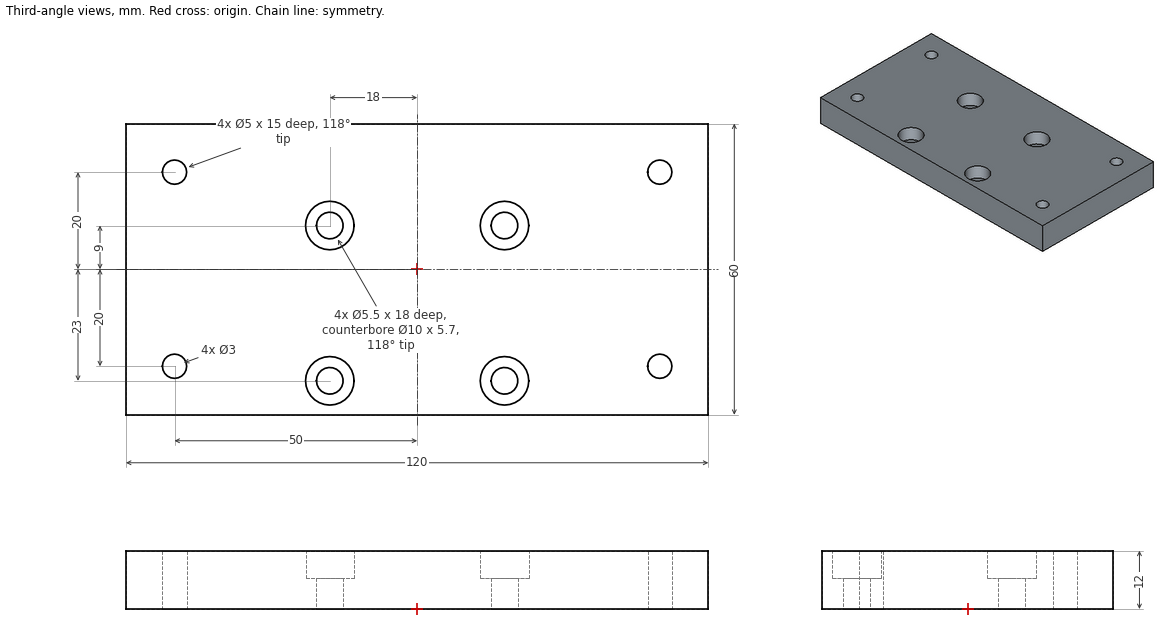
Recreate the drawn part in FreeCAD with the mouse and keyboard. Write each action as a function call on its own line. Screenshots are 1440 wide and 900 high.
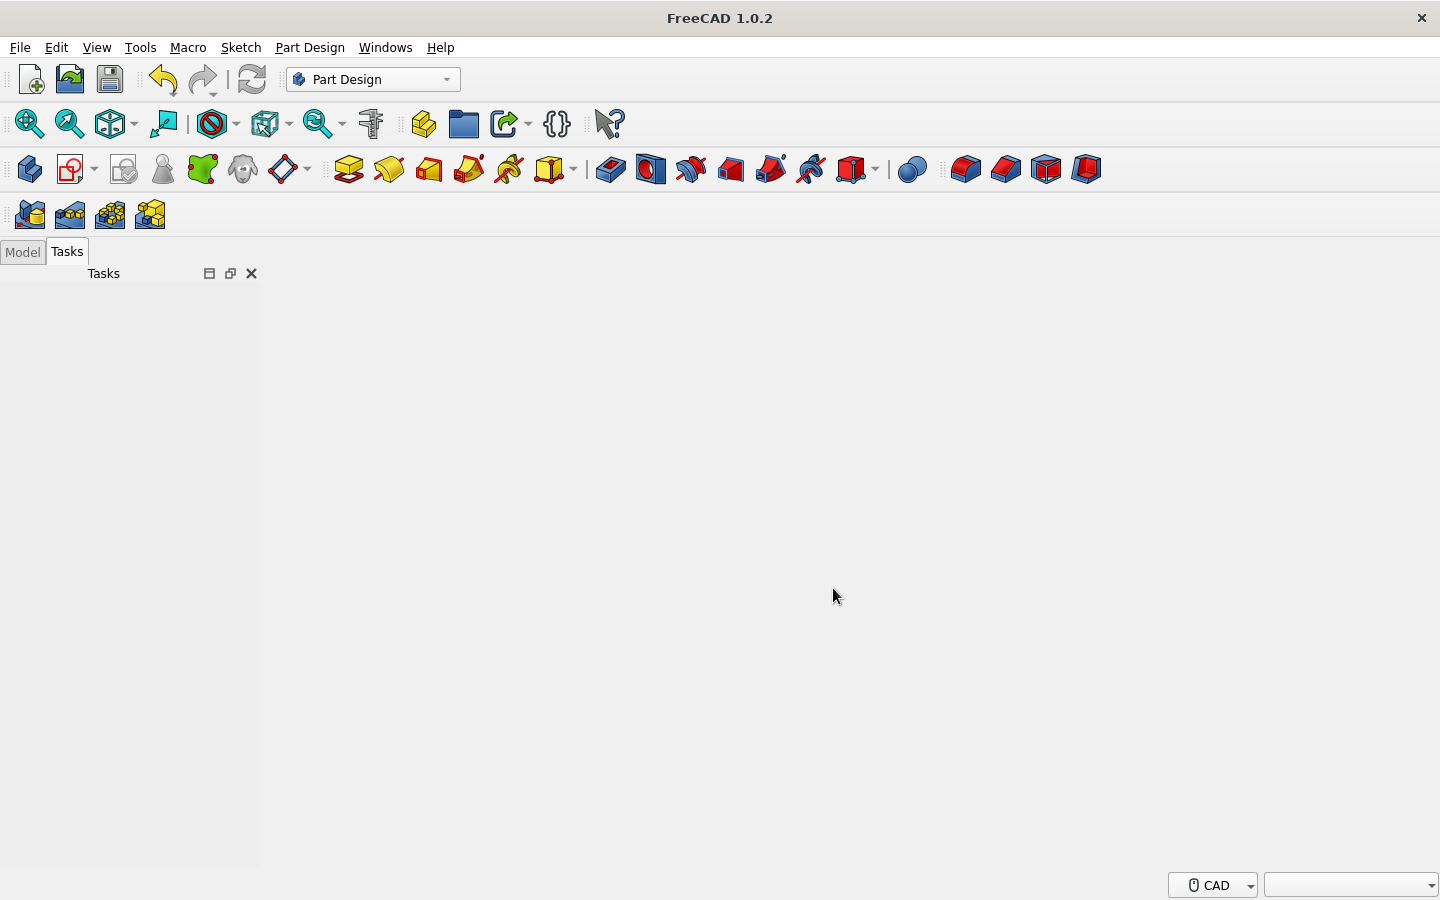
click(30, 80)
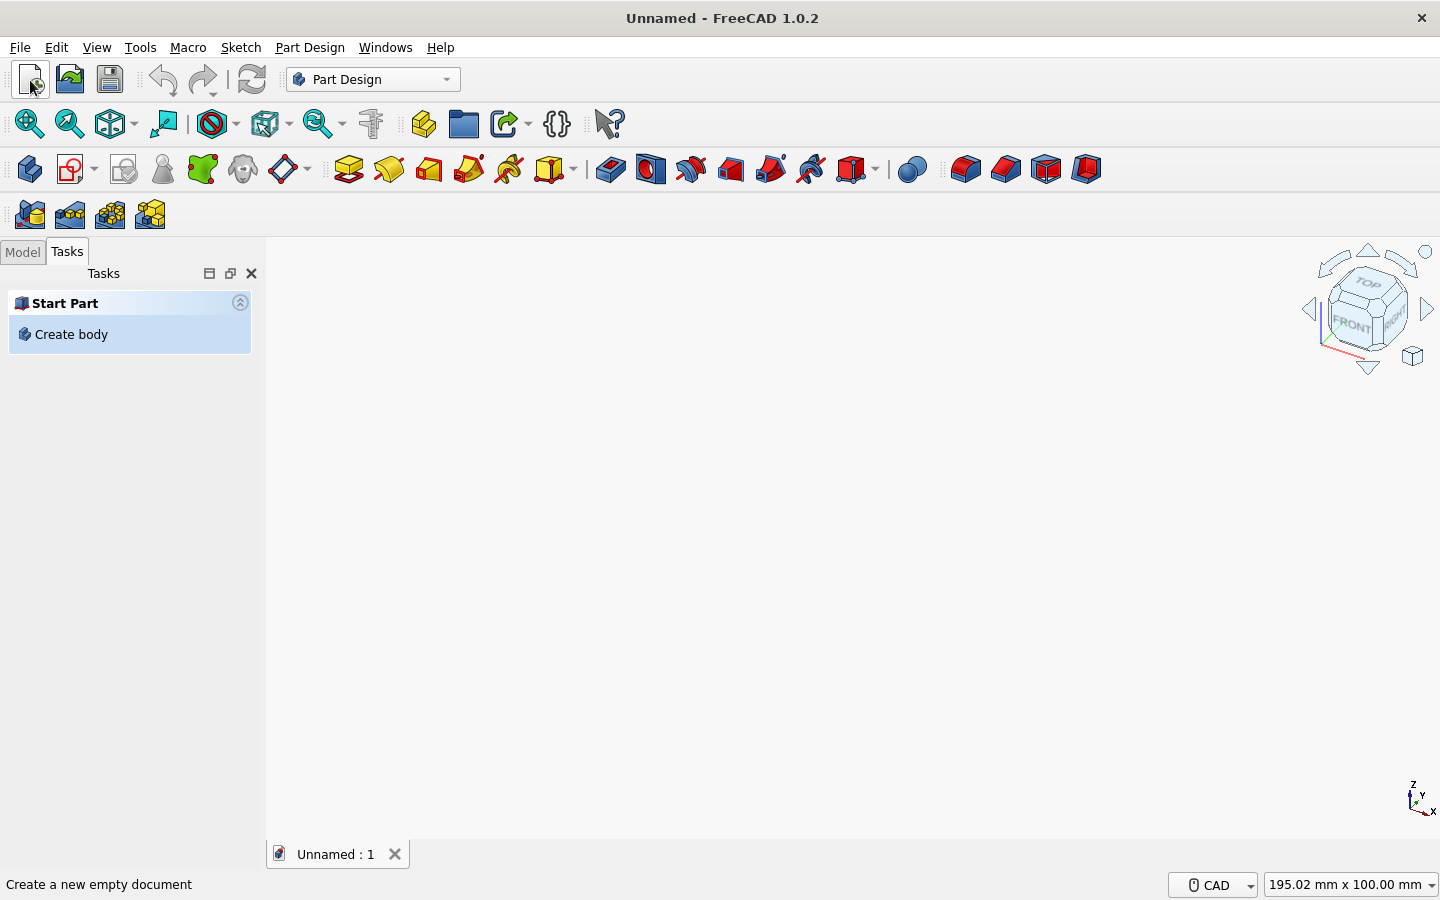
click(70, 170)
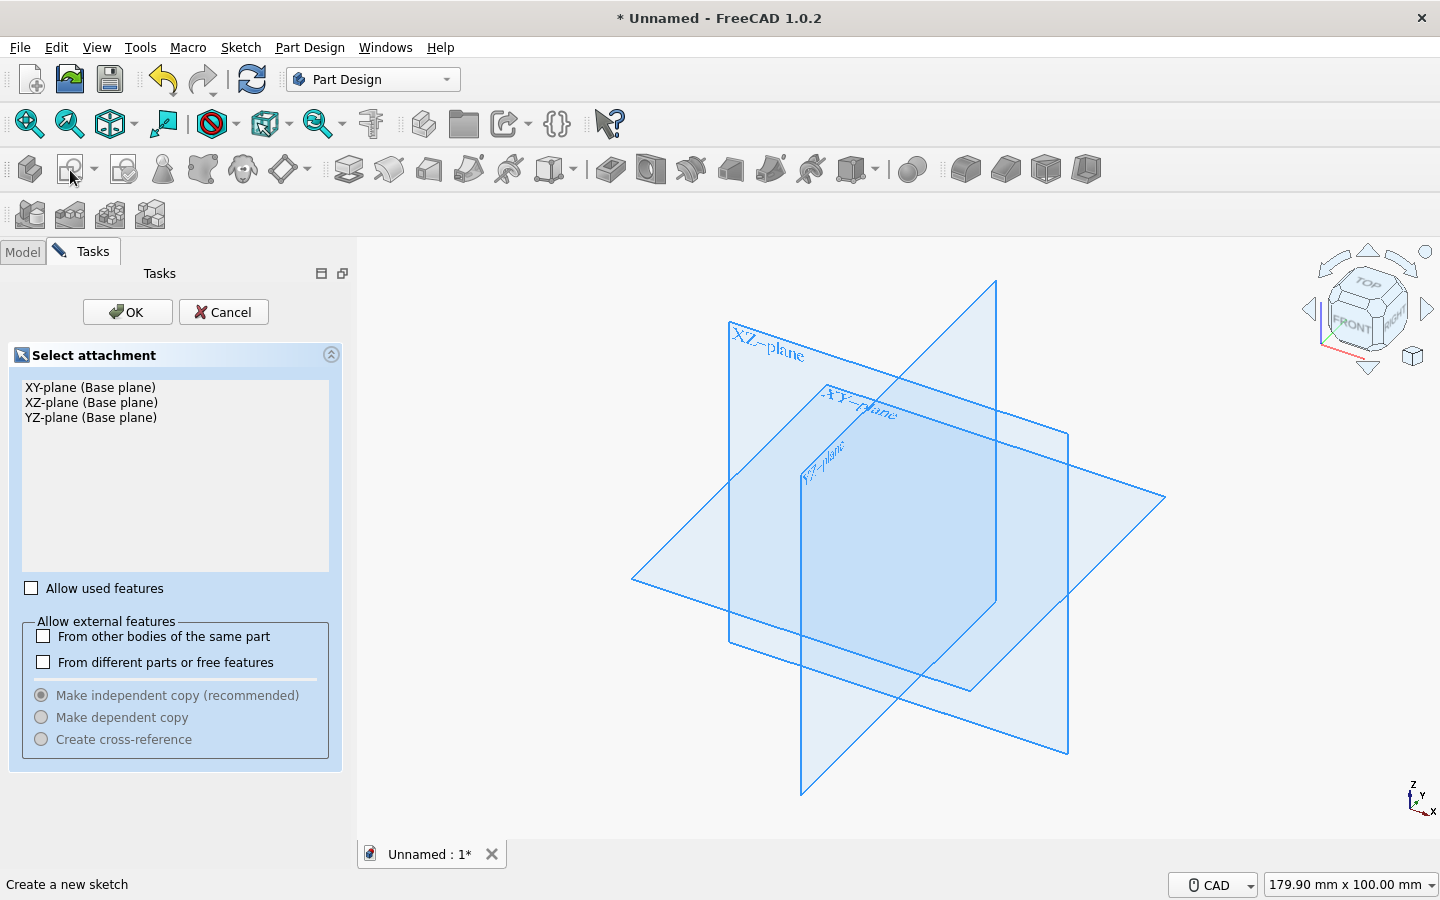
click(82, 388)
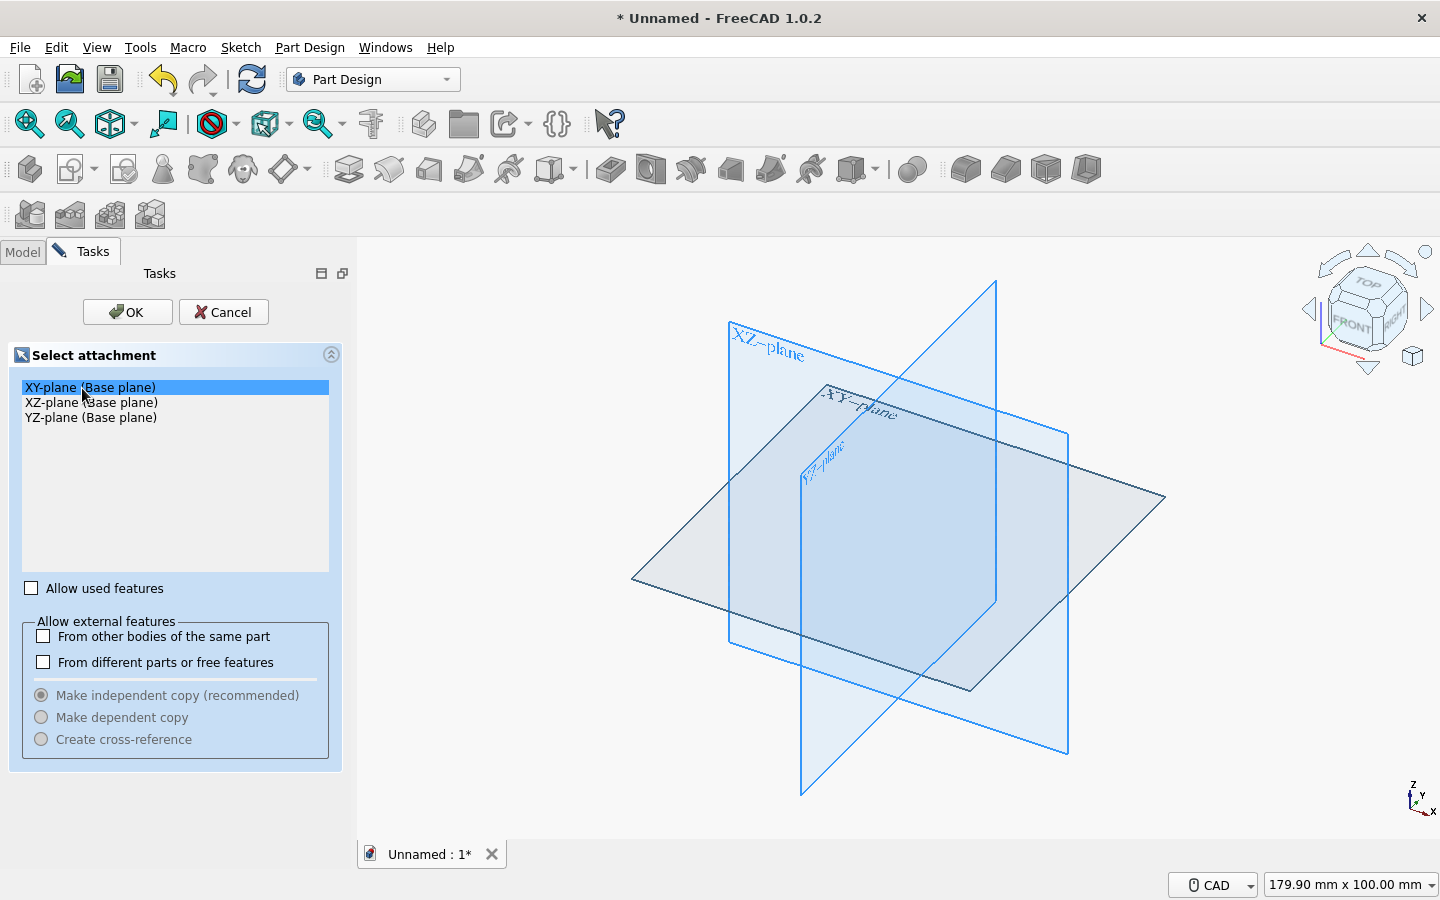
click(128, 312)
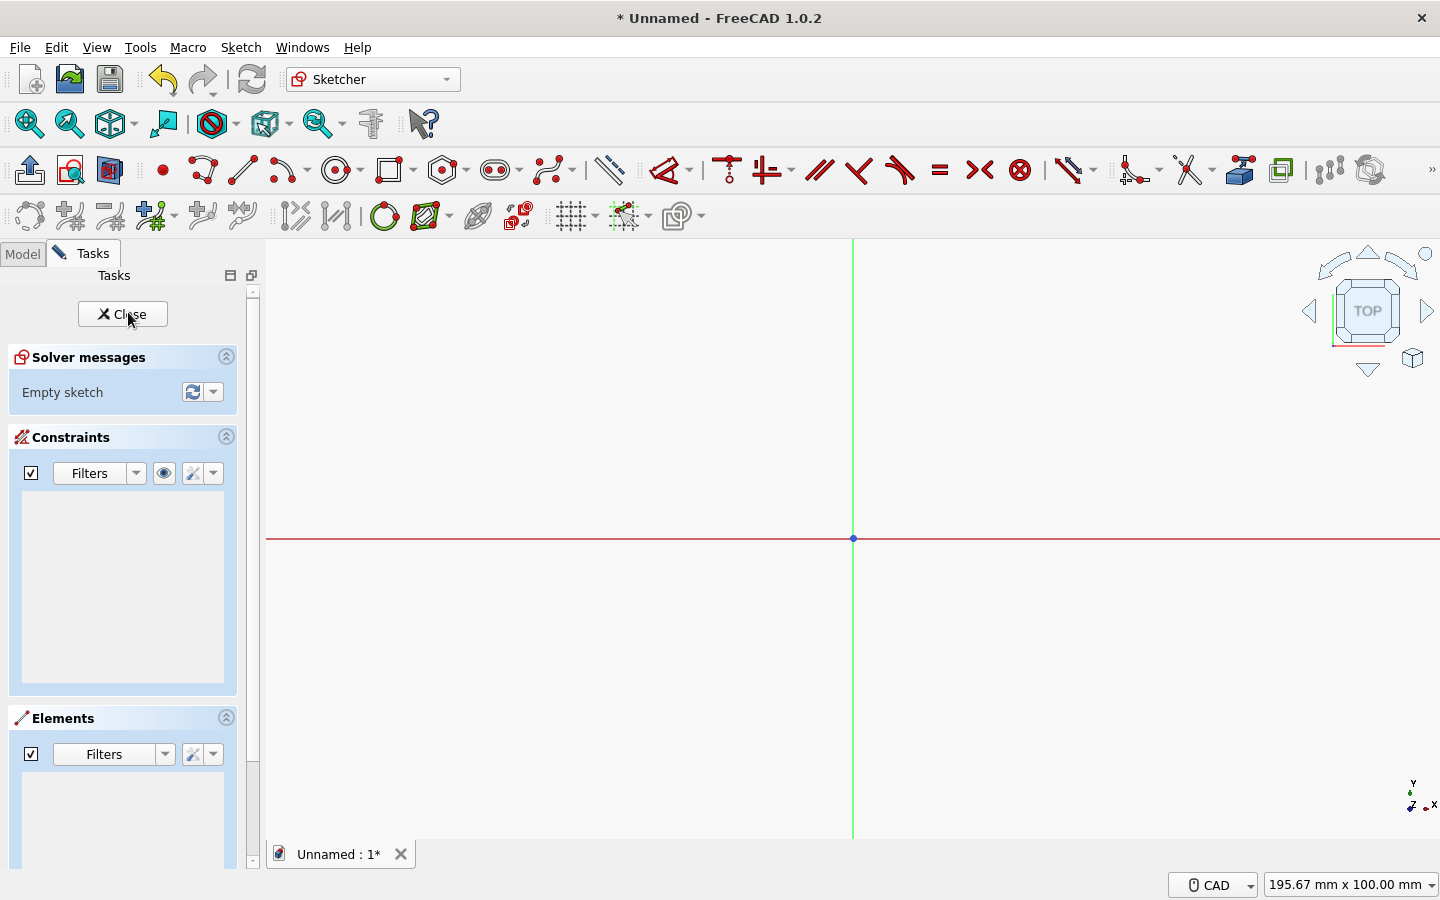
click(416, 170)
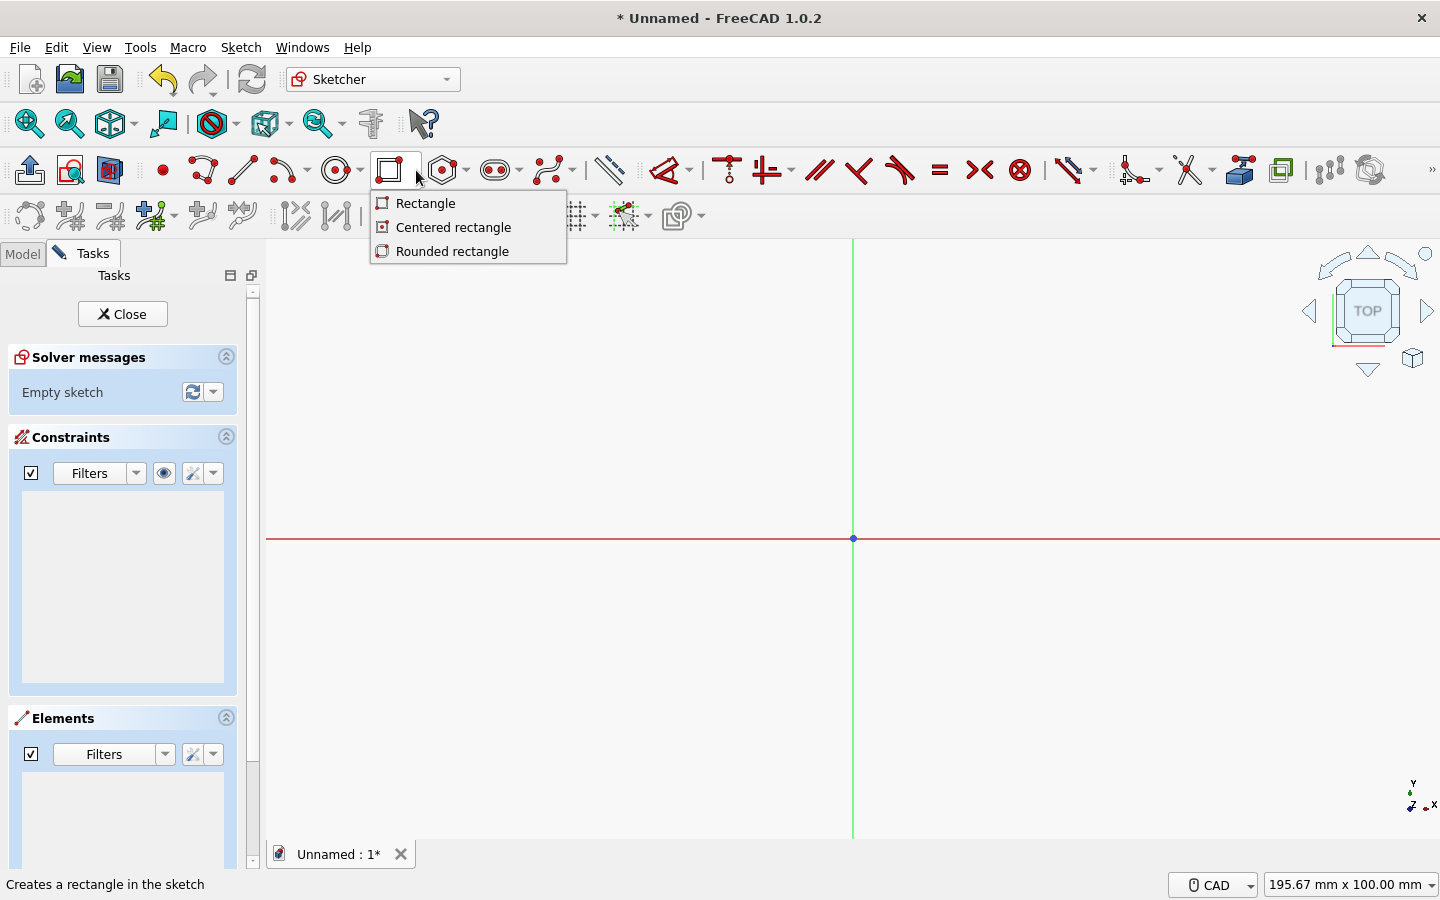
click(468, 227)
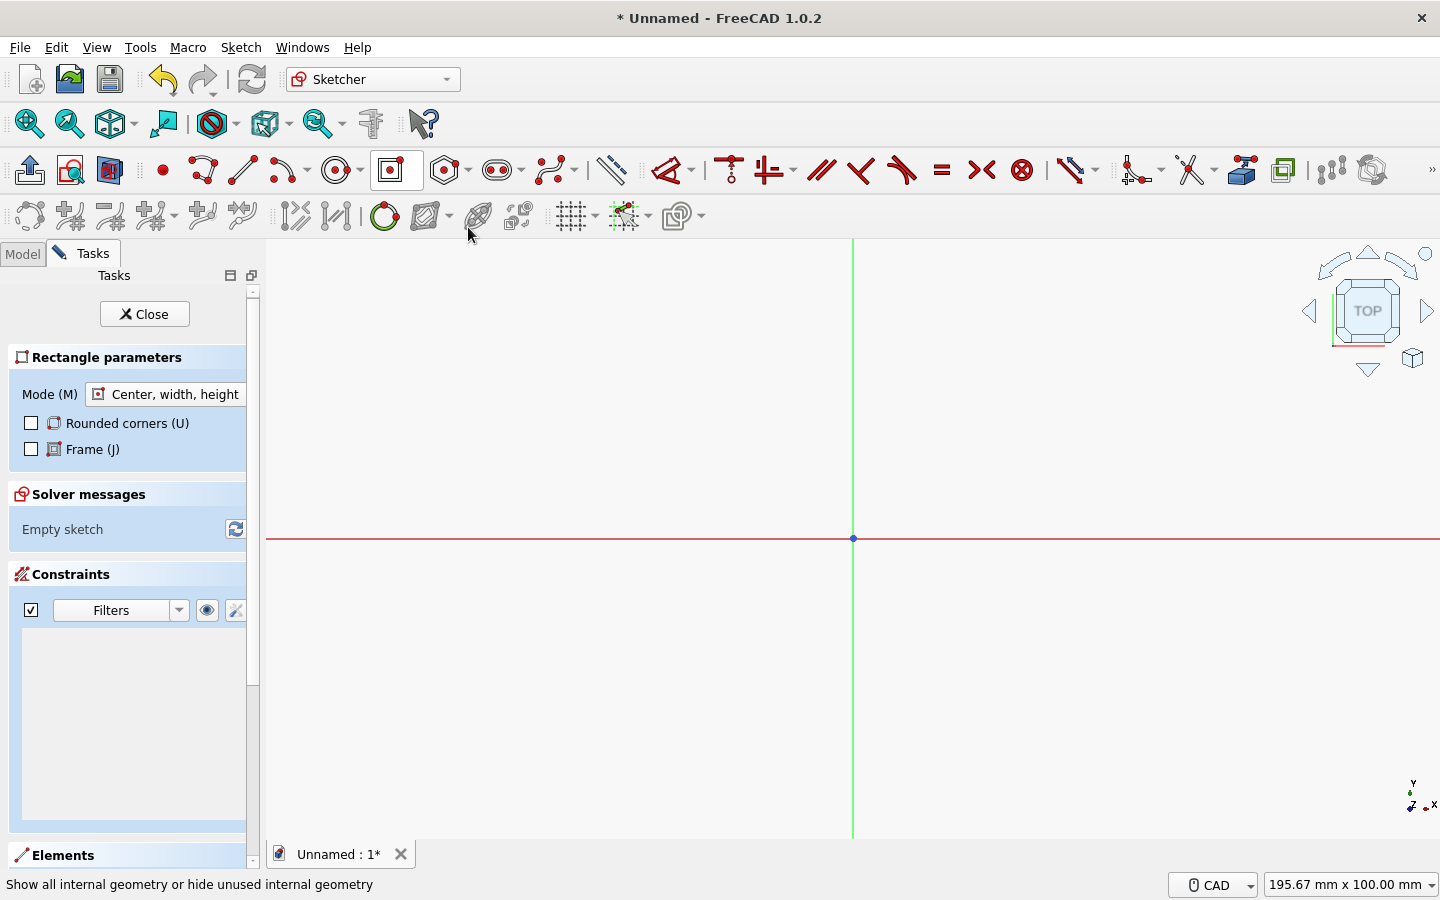
click(853, 539)
click(1213, 359)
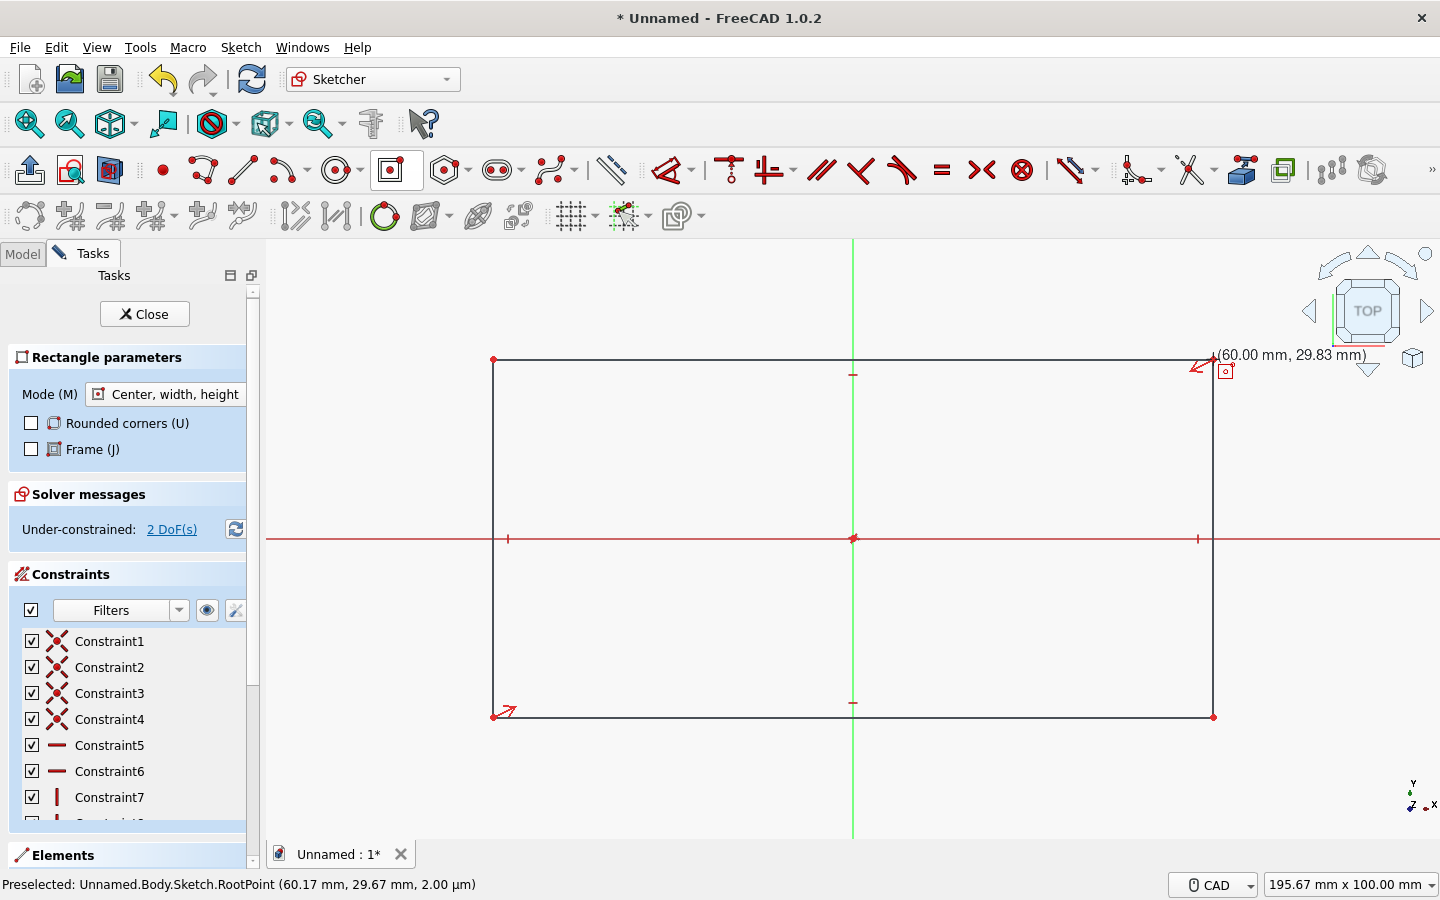
click(336, 170)